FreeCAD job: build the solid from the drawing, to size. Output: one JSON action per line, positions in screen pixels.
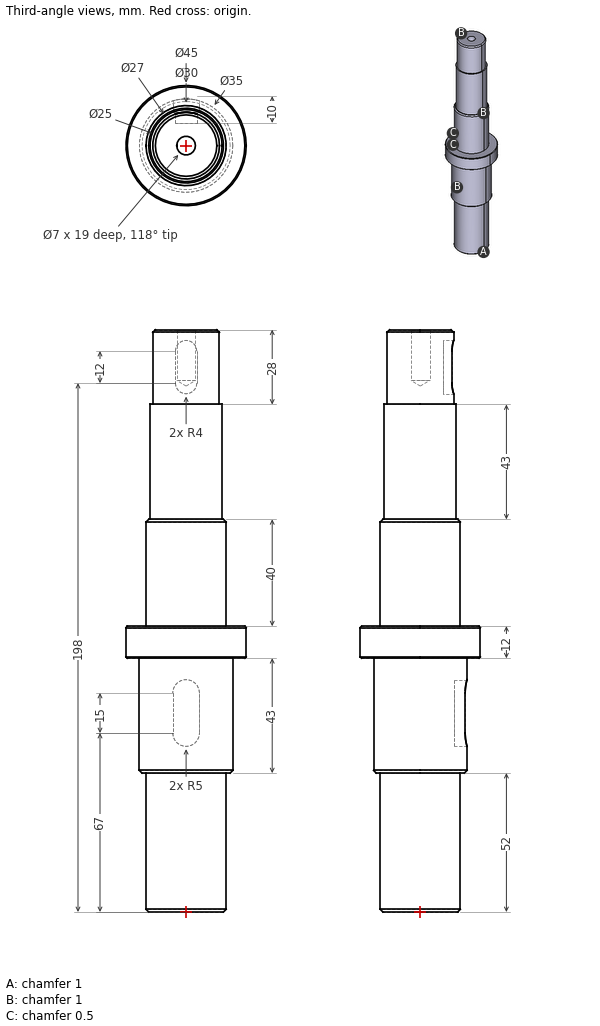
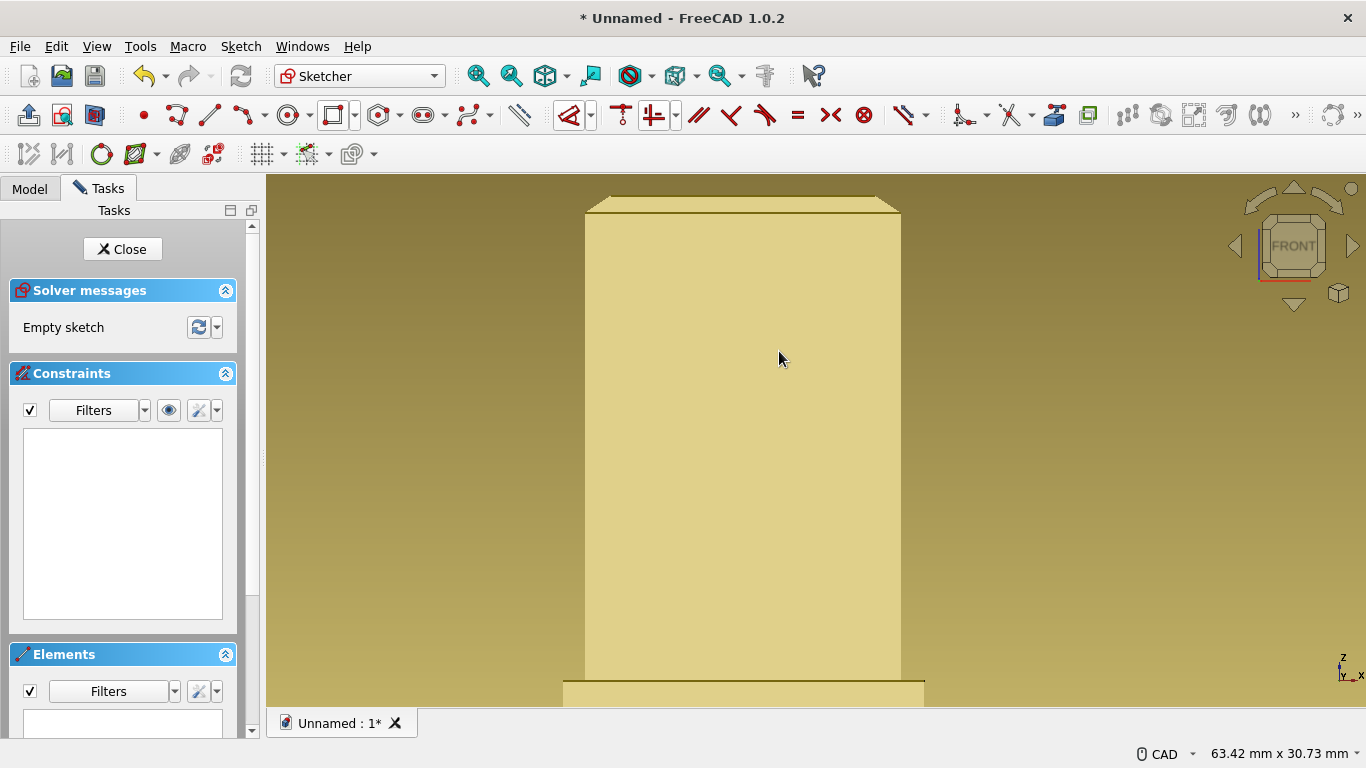
{"action": "key", "text": "g s"}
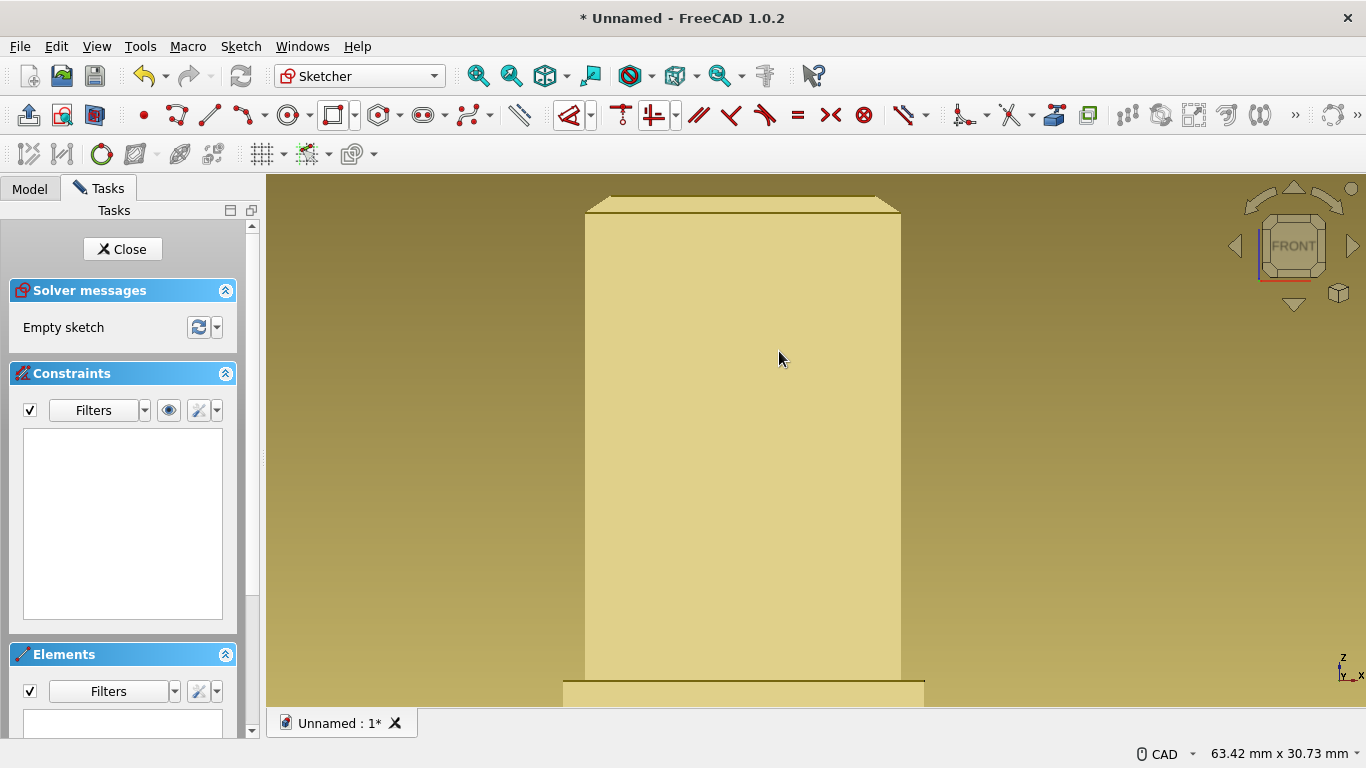
{"action": "left_click", "coordinate": [743, 543]}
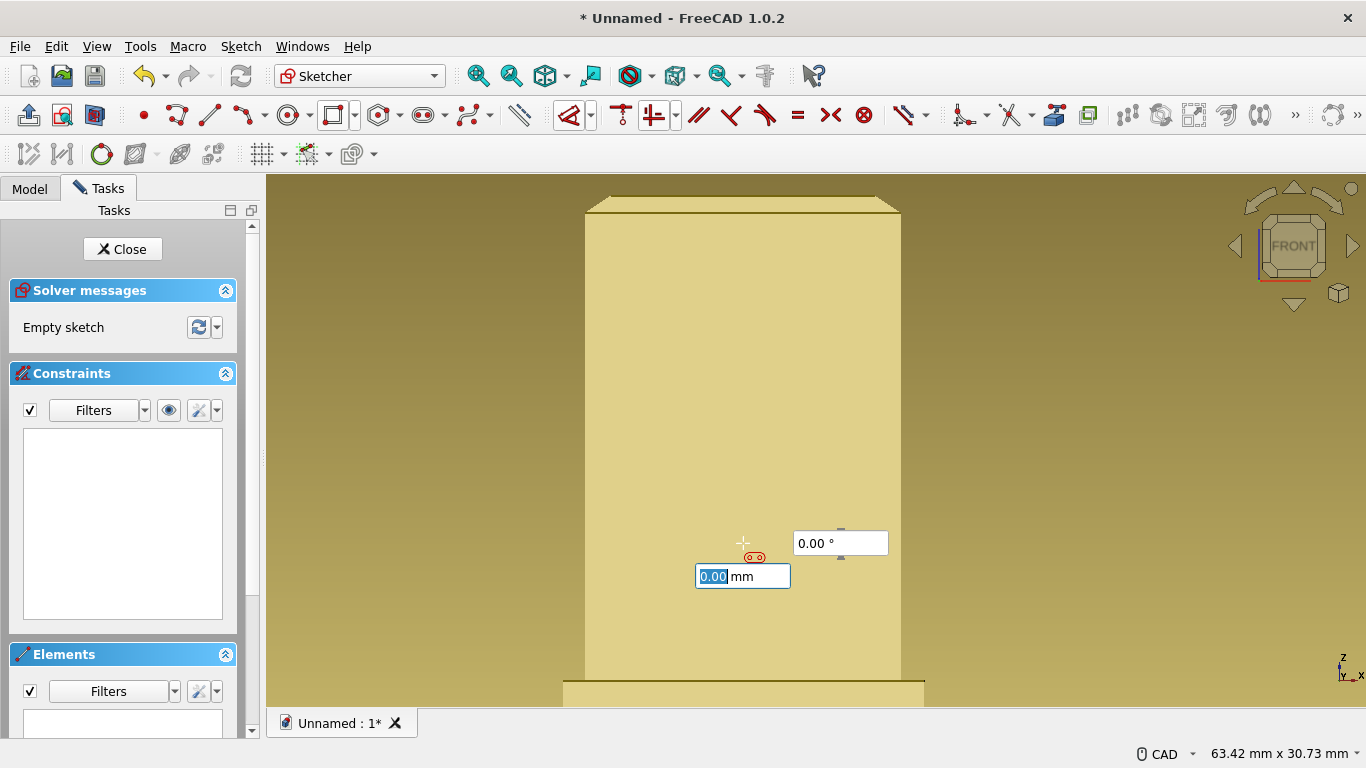
{"action": "left_click", "coordinate": [752, 334]}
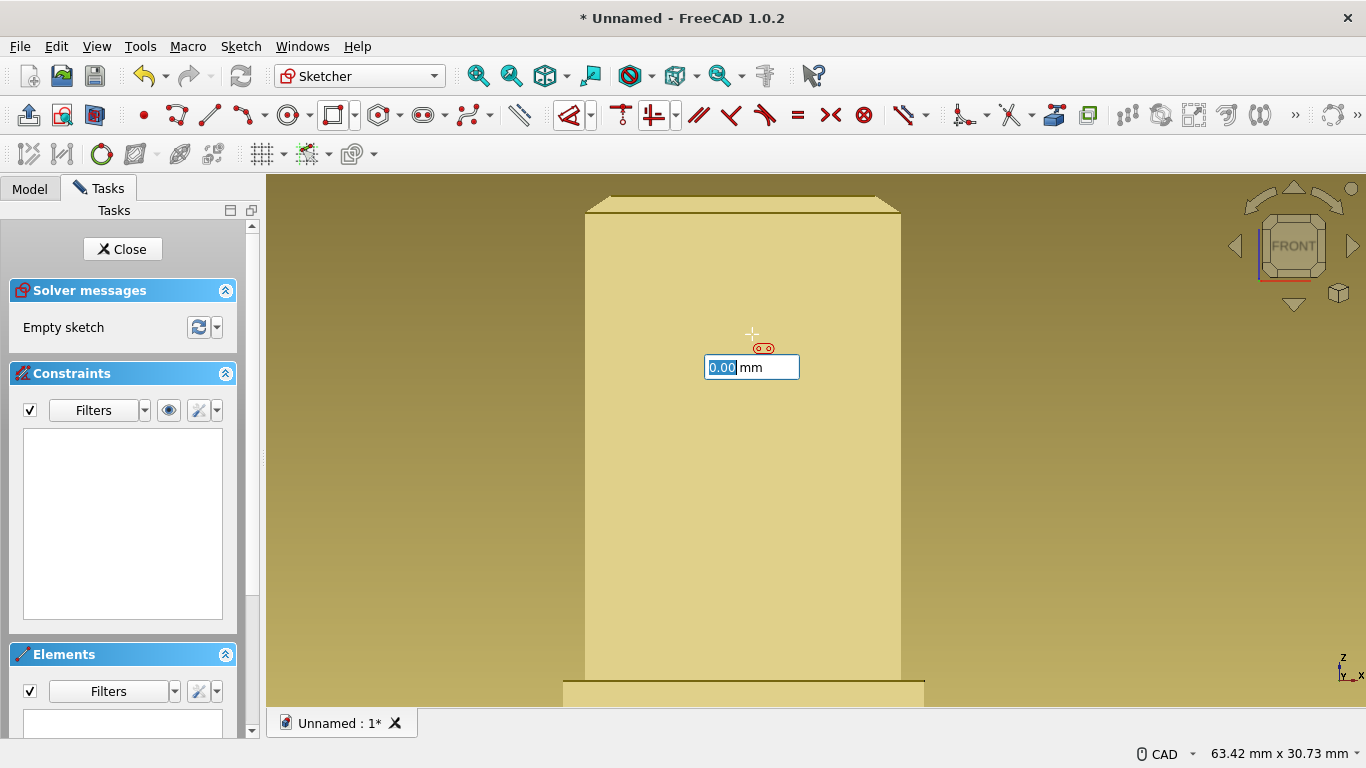
{"action": "left_click", "coordinate": [812, 439]}
{"action": "key", "text": "Escape"}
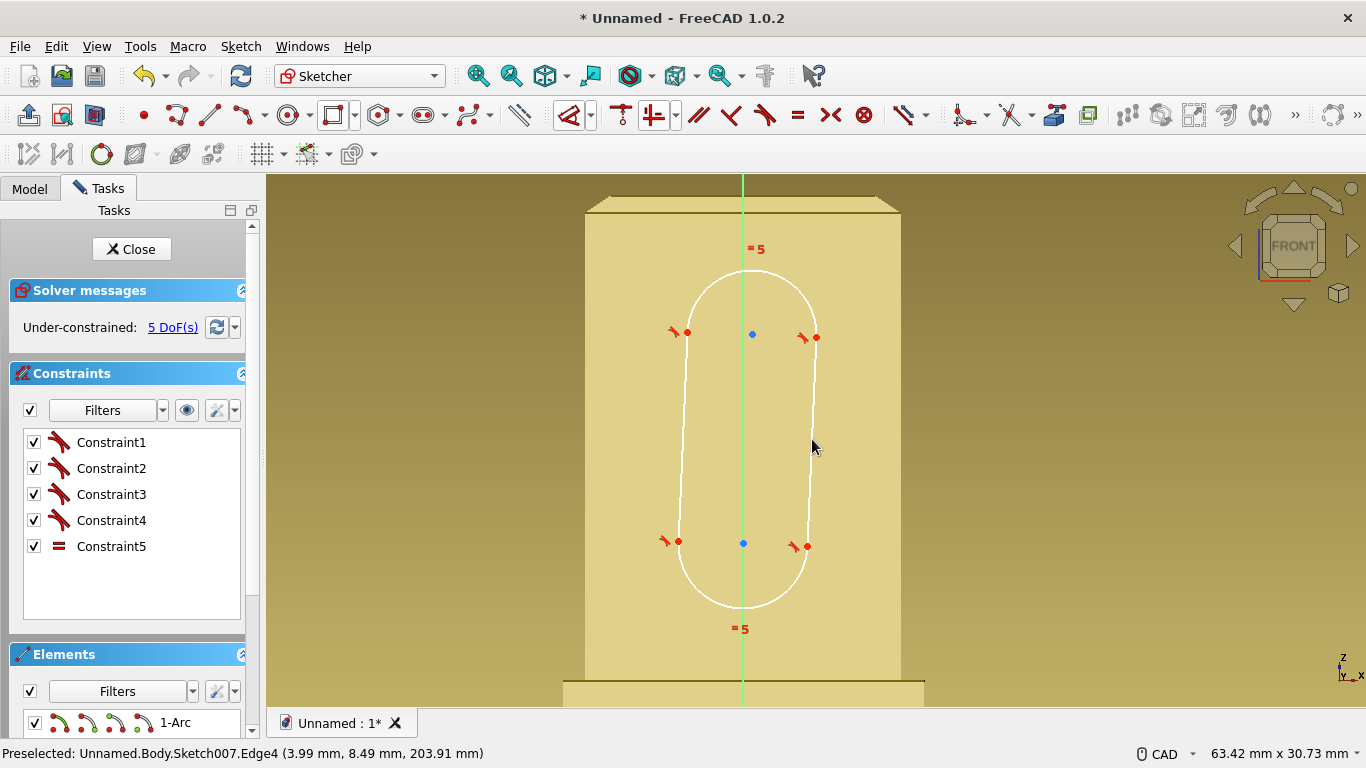
{"action": "left_click", "coordinate": [681, 479]}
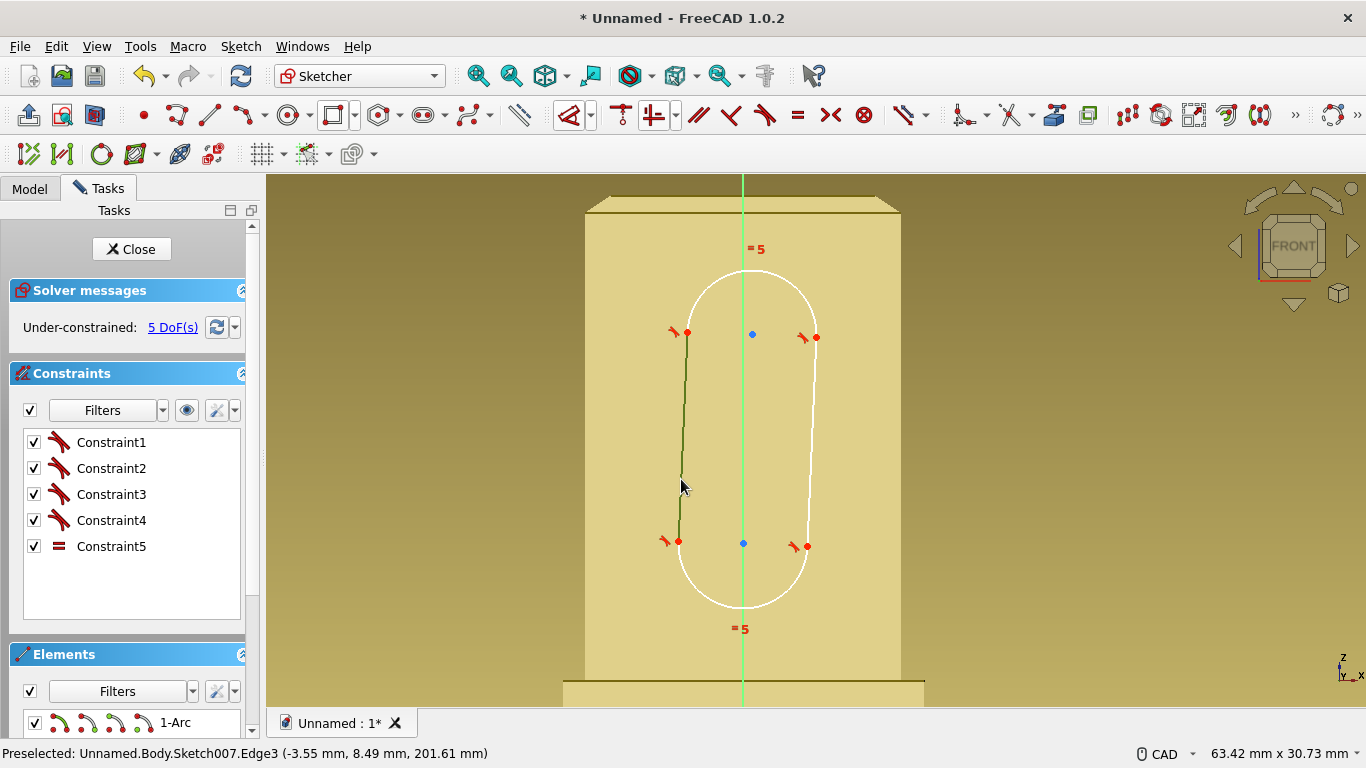
{"action": "key", "text": "v"}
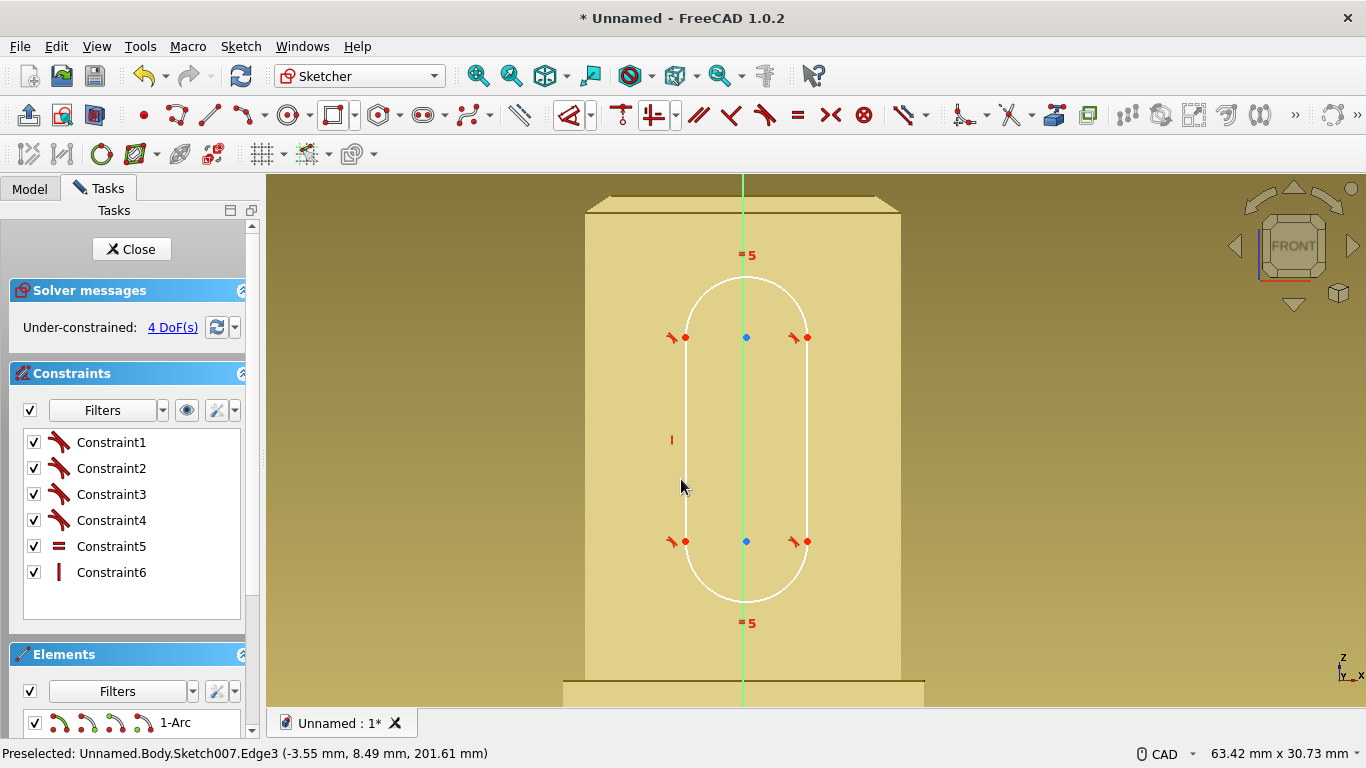
{"action": "left_click", "coordinate": [747, 541]}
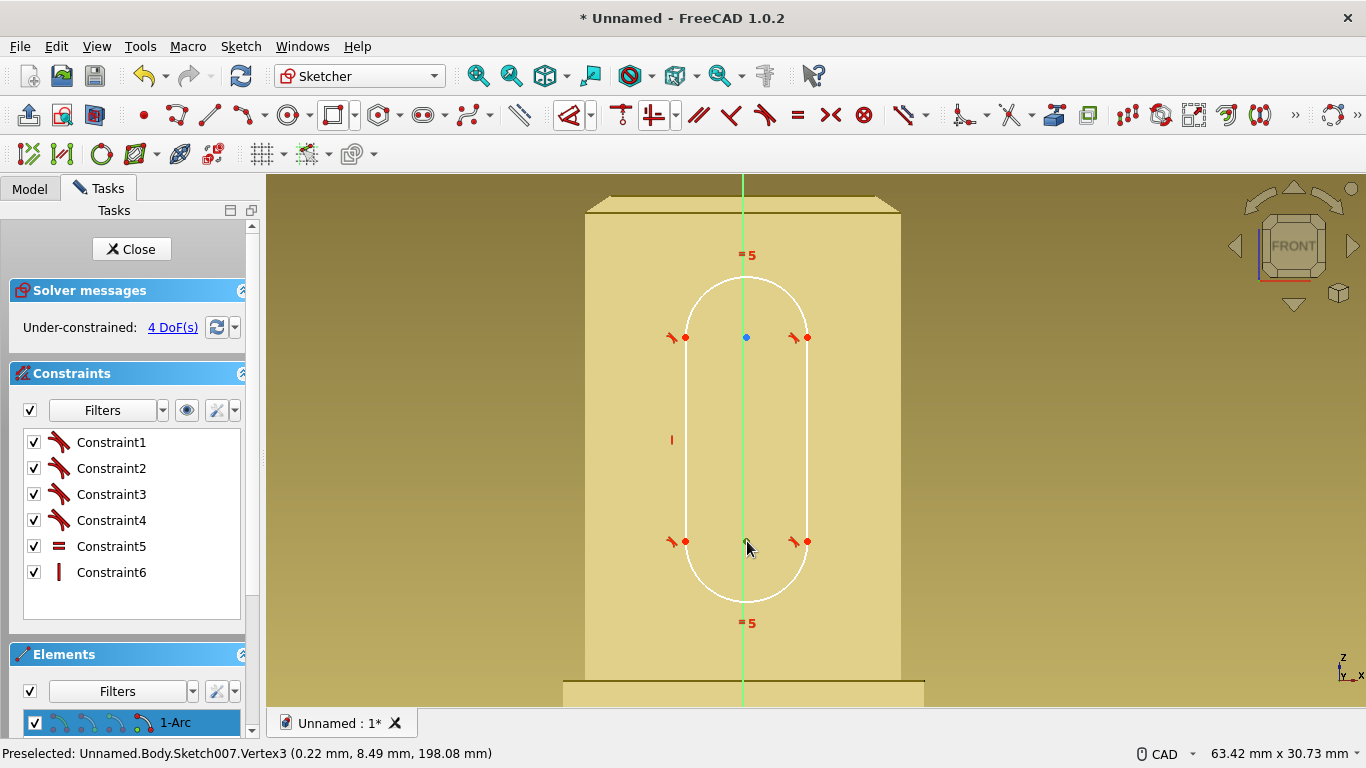
{"action": "left_click", "coordinate": [743, 645]}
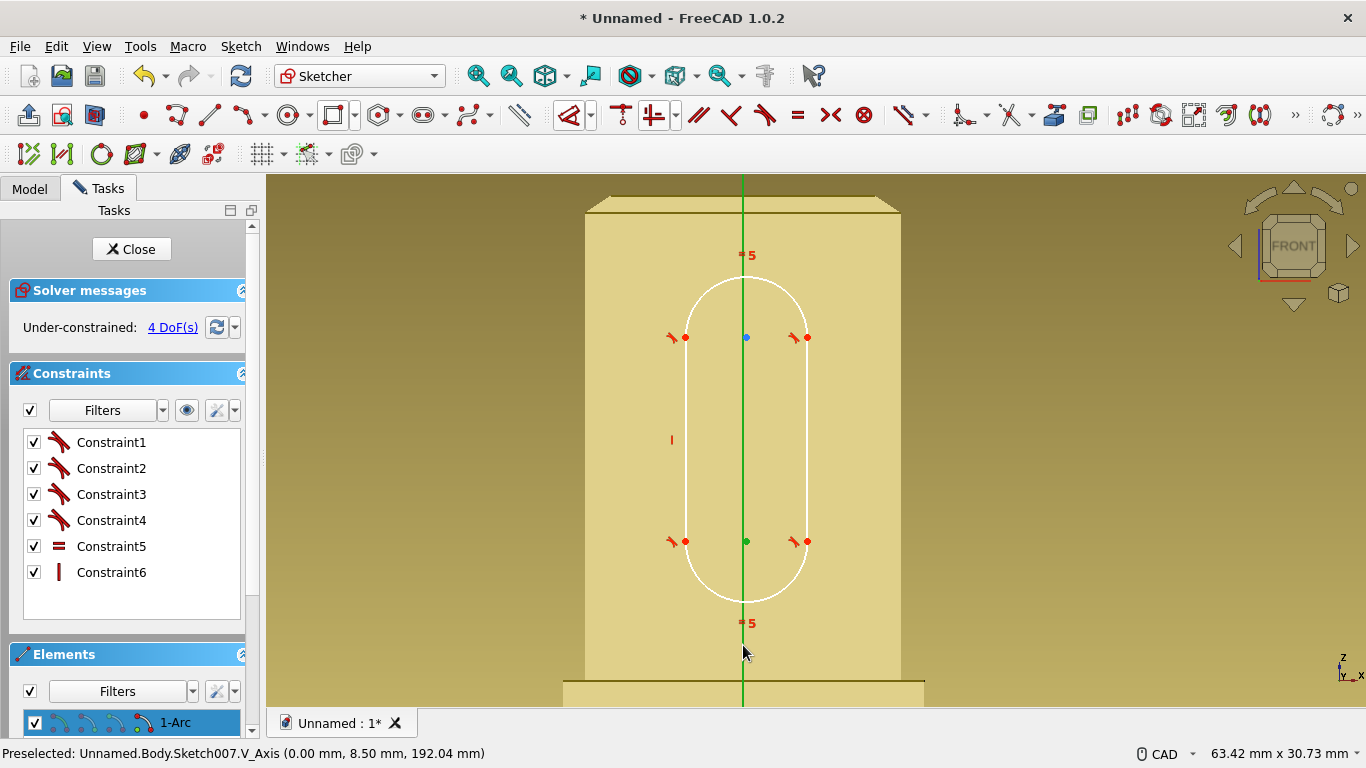
{"action": "key", "text": "c"}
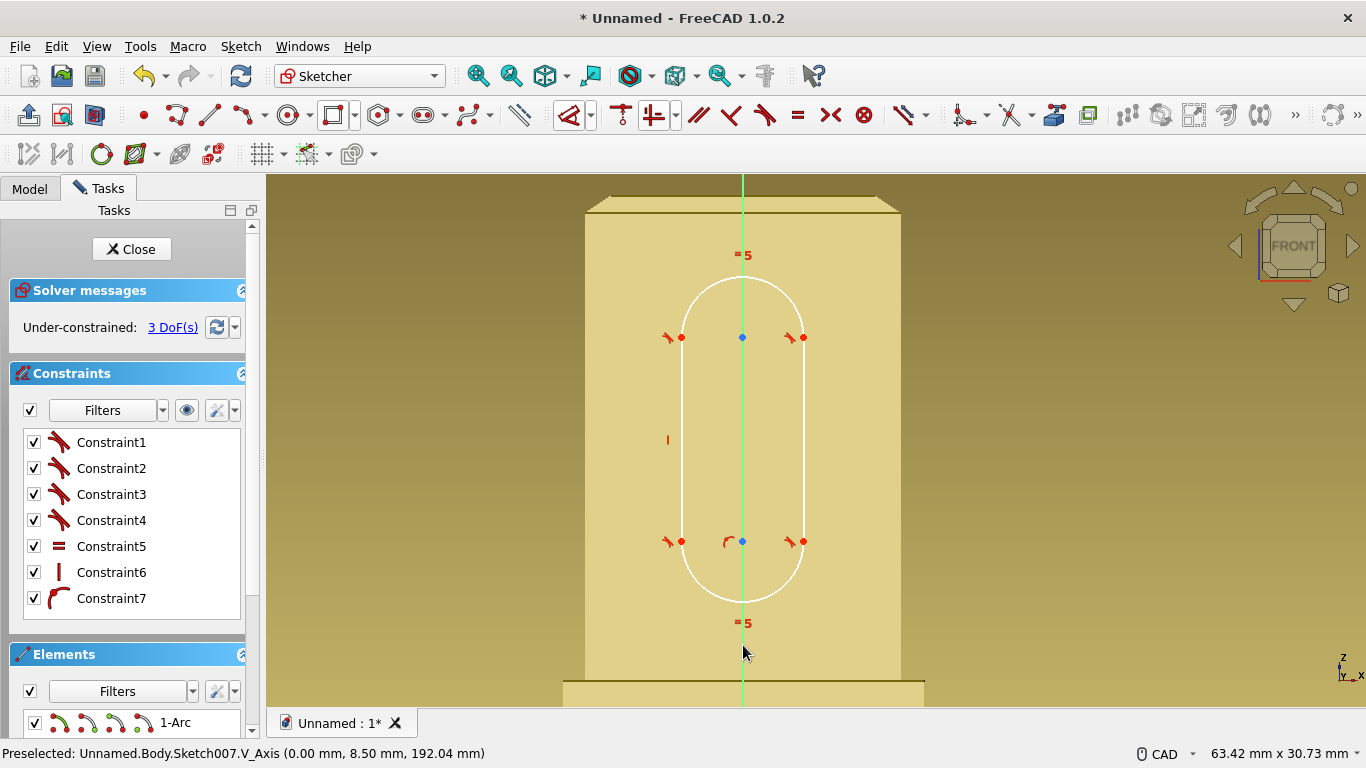
{"action": "left_click", "coordinate": [707, 590]}